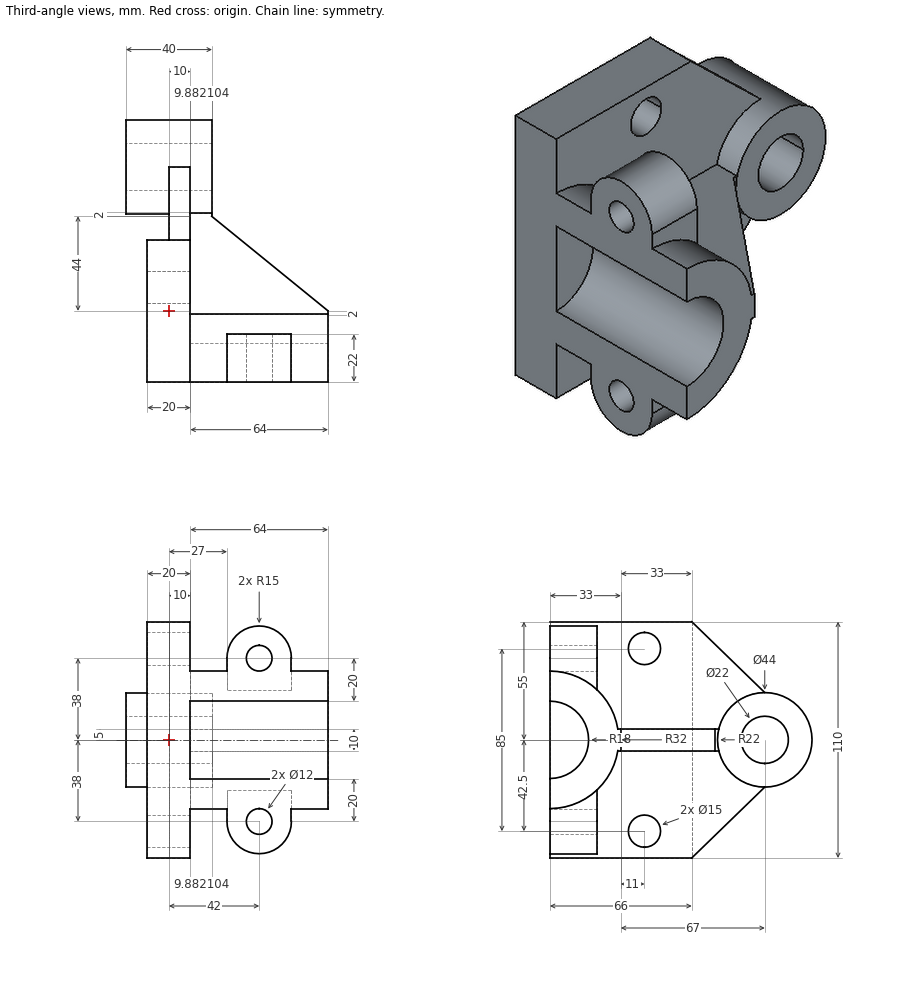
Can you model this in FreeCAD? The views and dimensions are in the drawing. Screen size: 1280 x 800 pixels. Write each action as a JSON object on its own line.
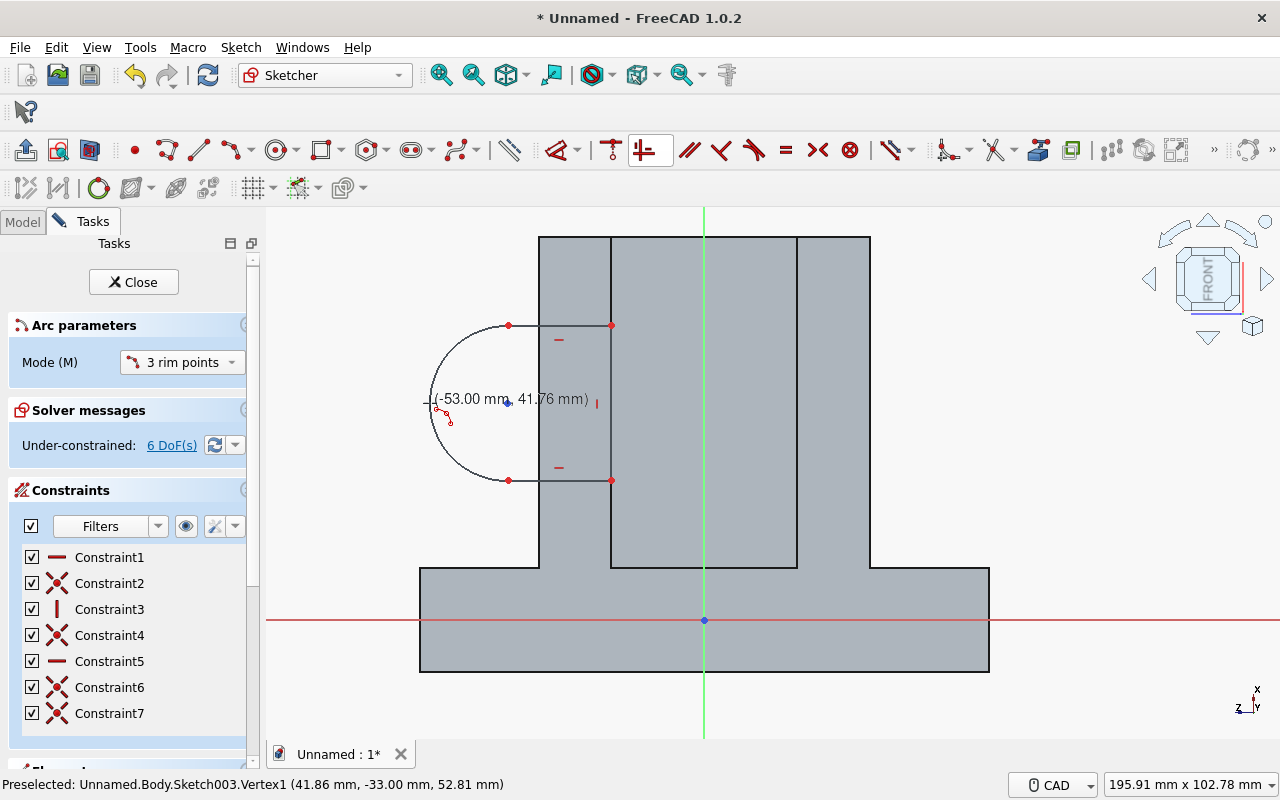
{"action": "left_click", "coordinate": [168, 150]}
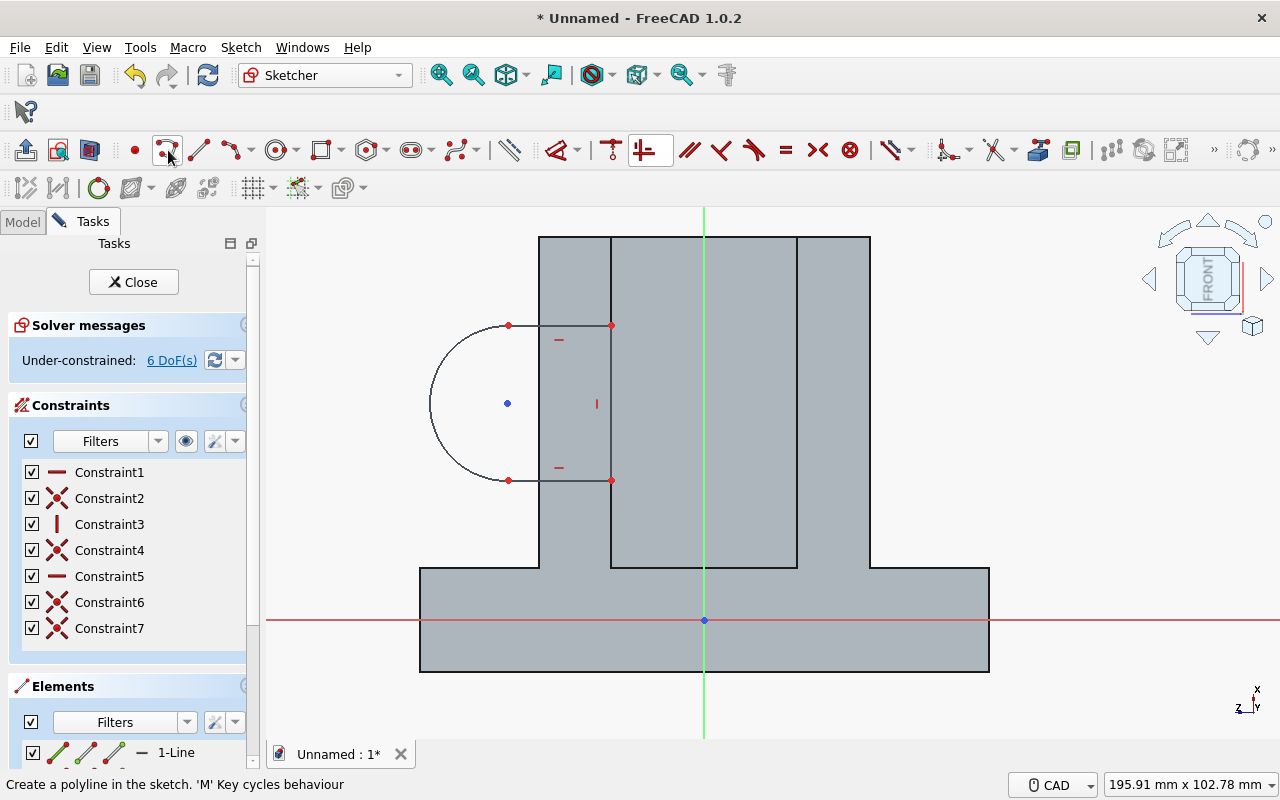
{"action": "left_click", "coordinate": [901, 325]}
{"action": "left_click", "coordinate": [797, 325]}
{"action": "left_click", "coordinate": [797, 480]}
{"action": "left_click", "coordinate": [901, 480]}
{"action": "right_click", "coordinate": [901, 480]}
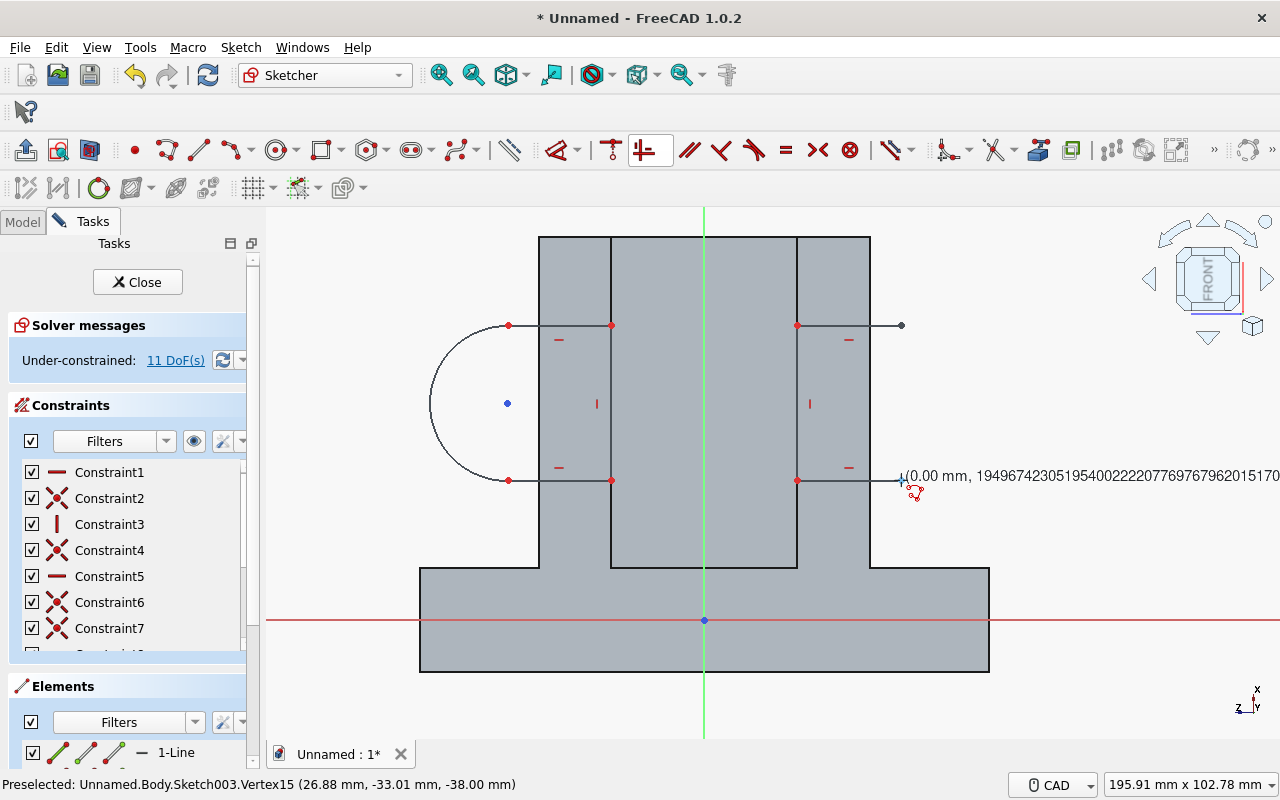
{"action": "left_click", "coordinate": [232, 150]}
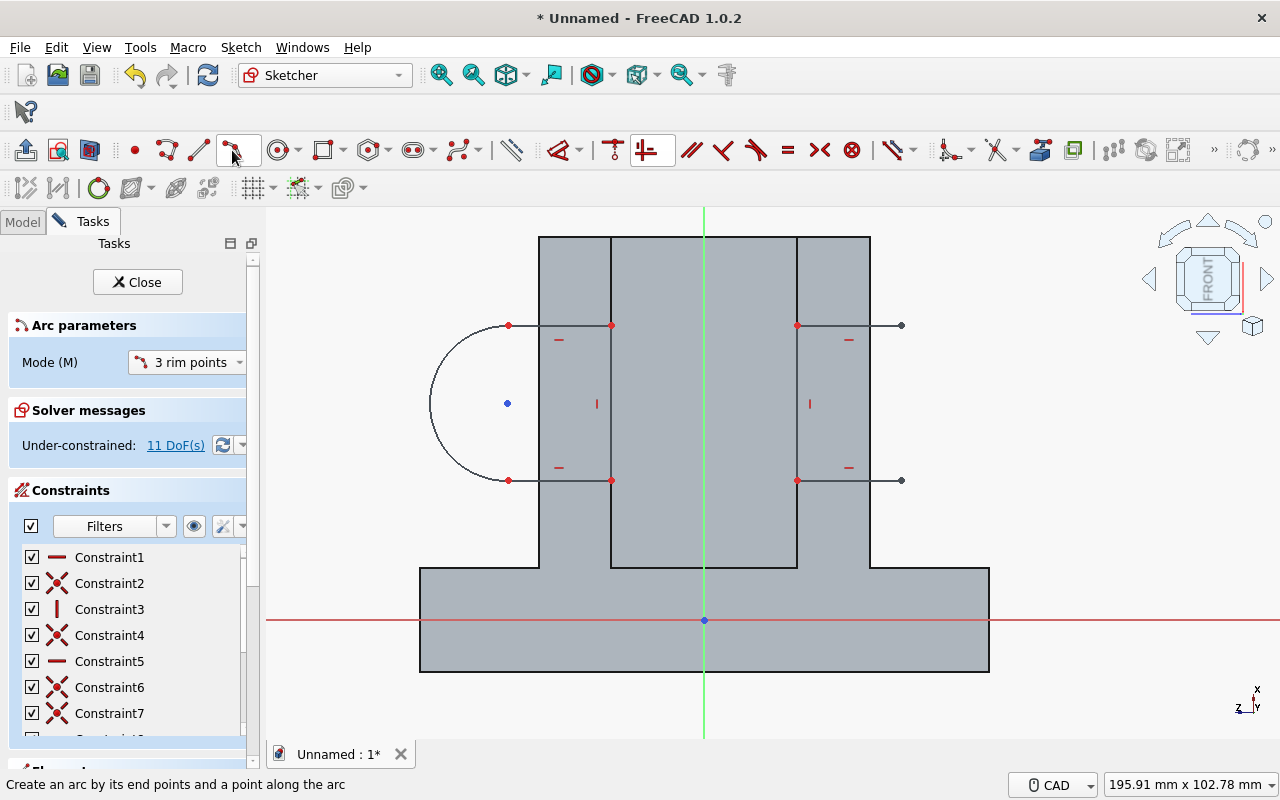
{"action": "left_click", "coordinate": [901, 481]}
{"action": "left_click", "coordinate": [901, 326]}
{"action": "left_click", "coordinate": [979, 403]}
{"action": "key", "text": "Escape"}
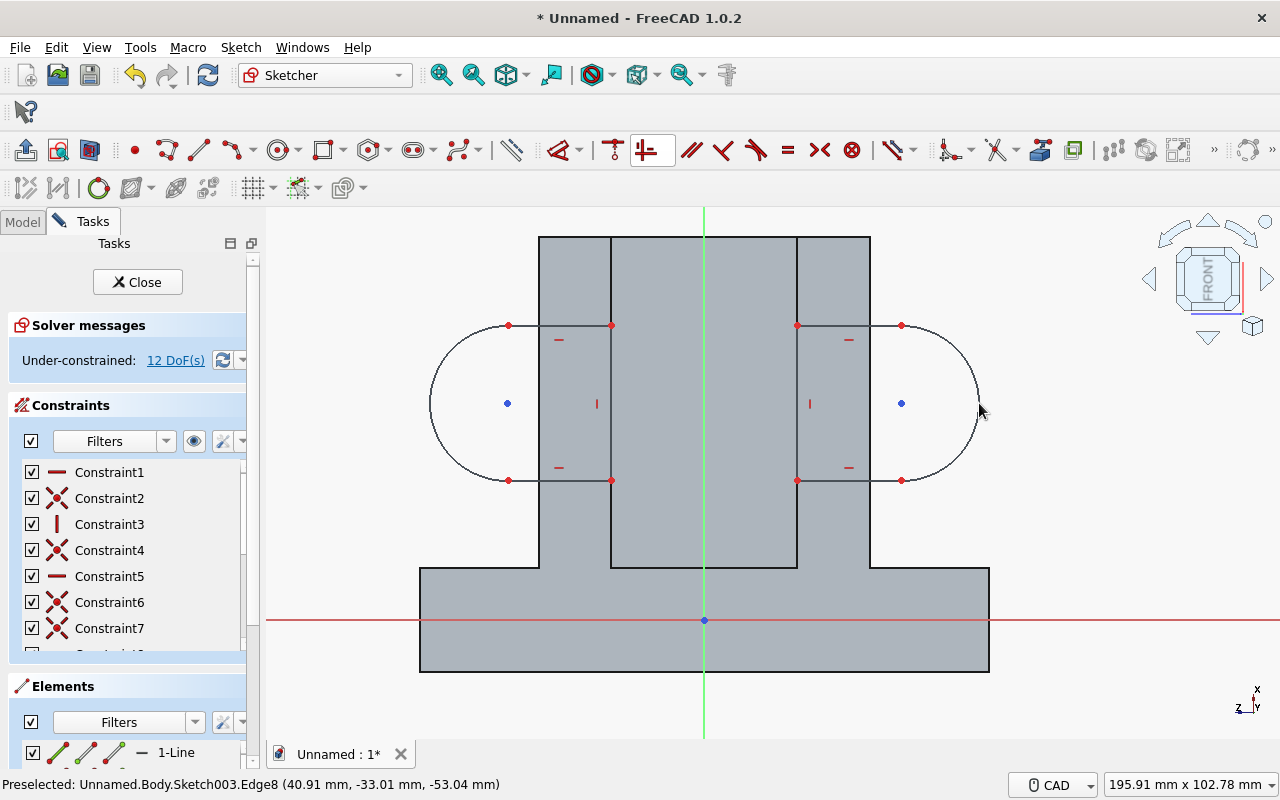
{"action": "left_click", "coordinate": [539, 481]}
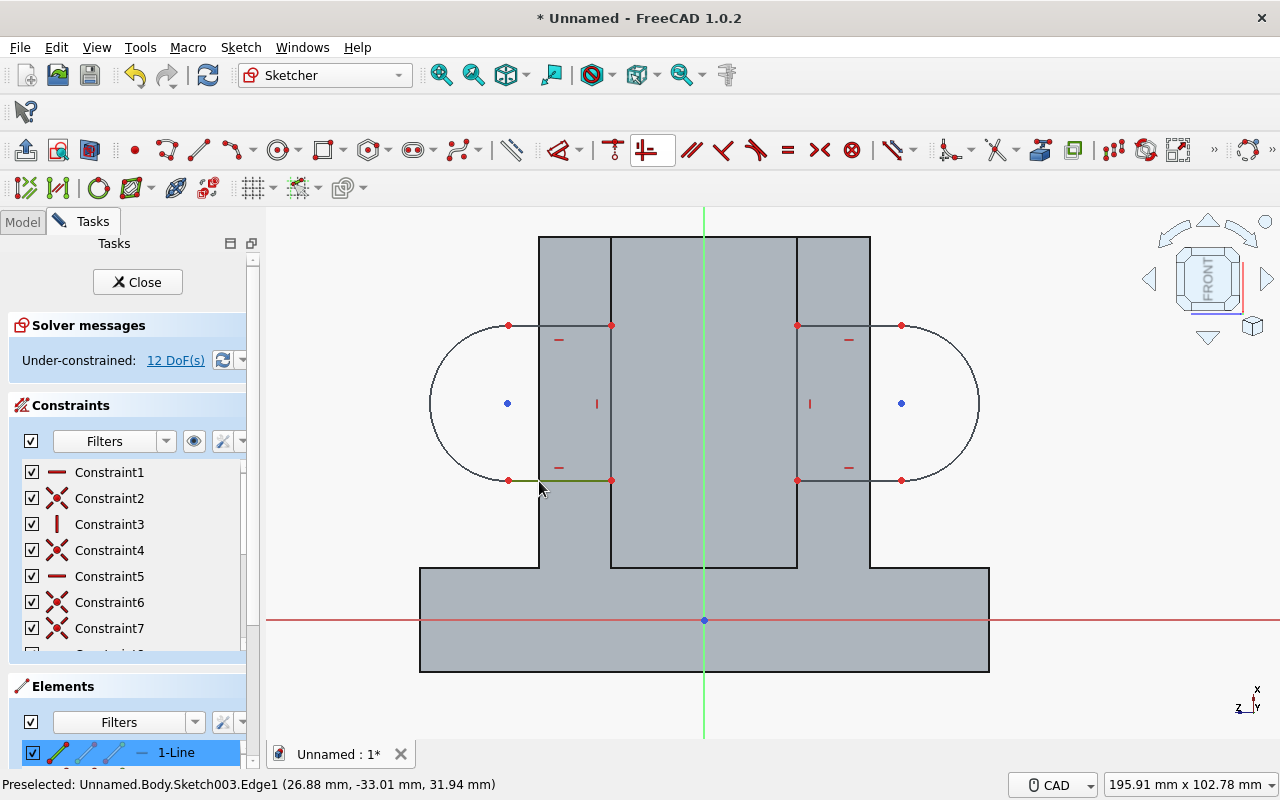
{"action": "left_click", "coordinate": [445, 358]}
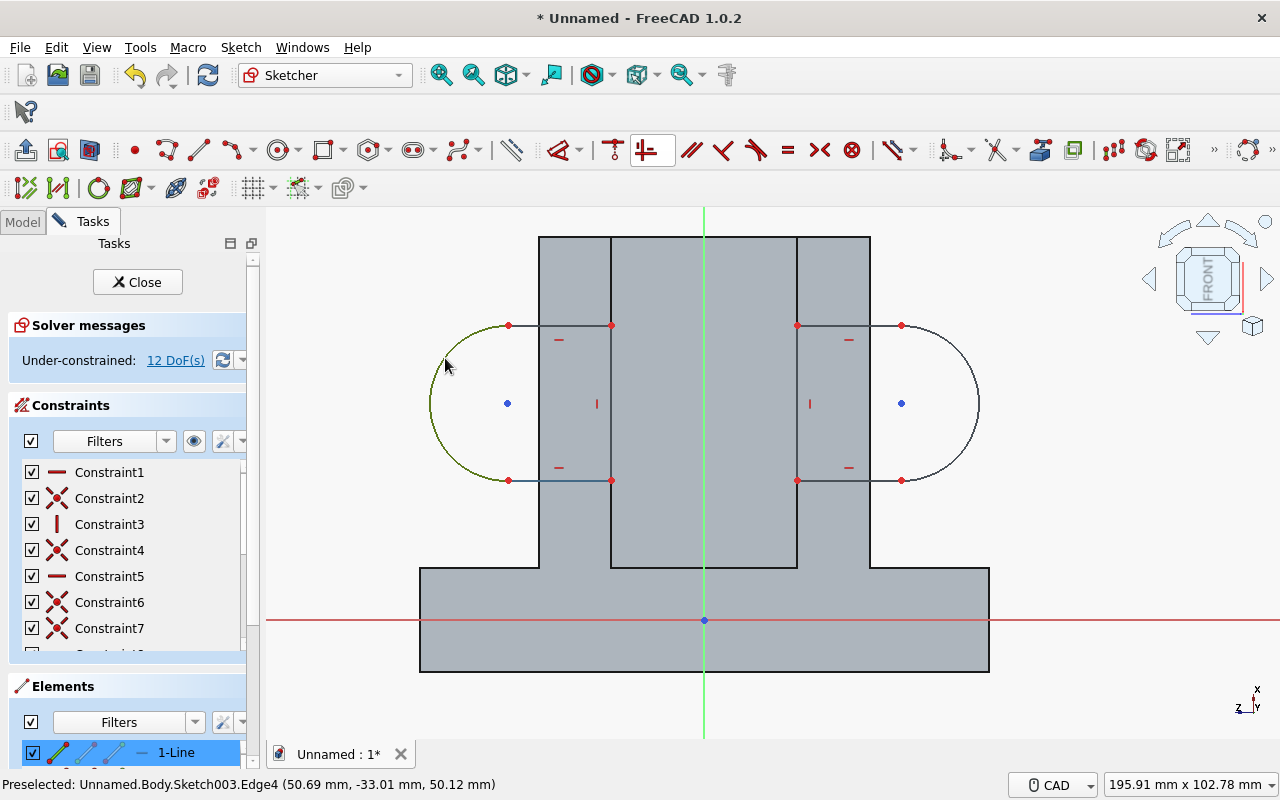
{"action": "left_click", "coordinate": [756, 150]}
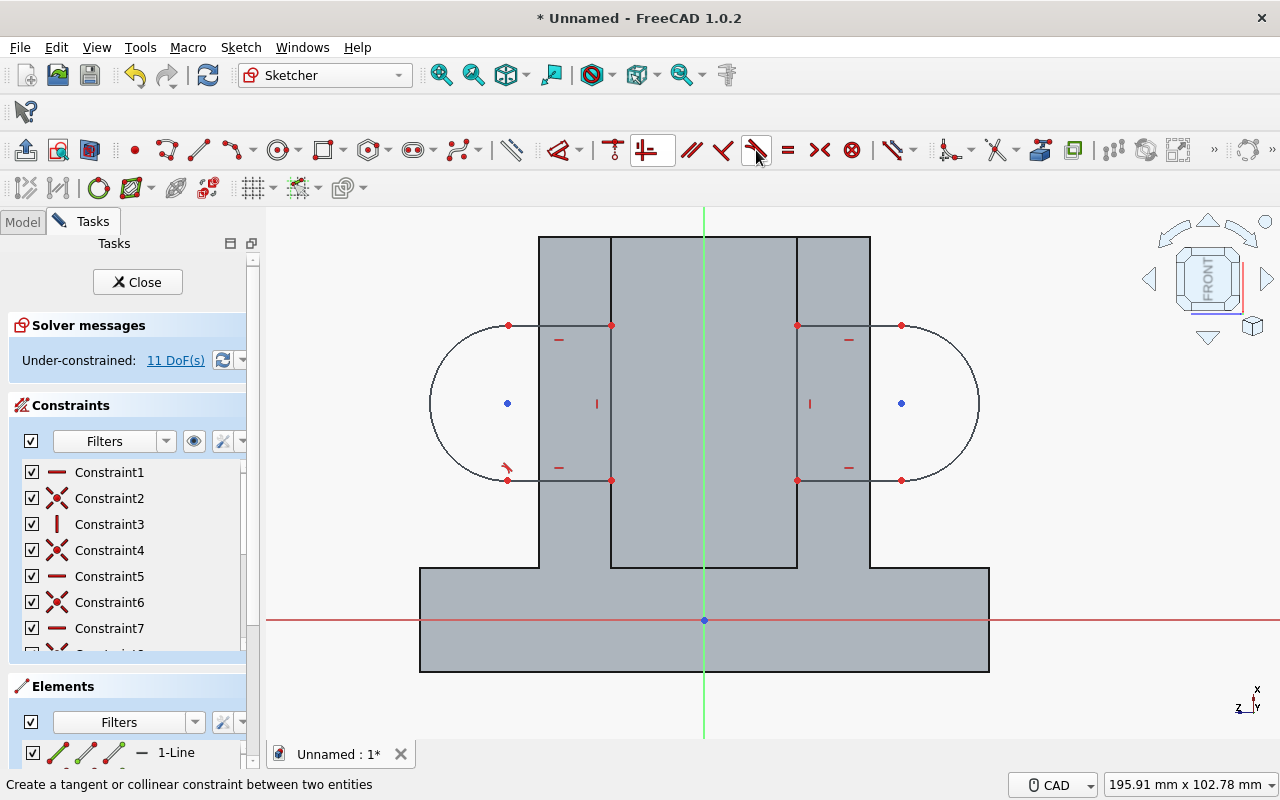
{"action": "left_click", "coordinate": [580, 326]}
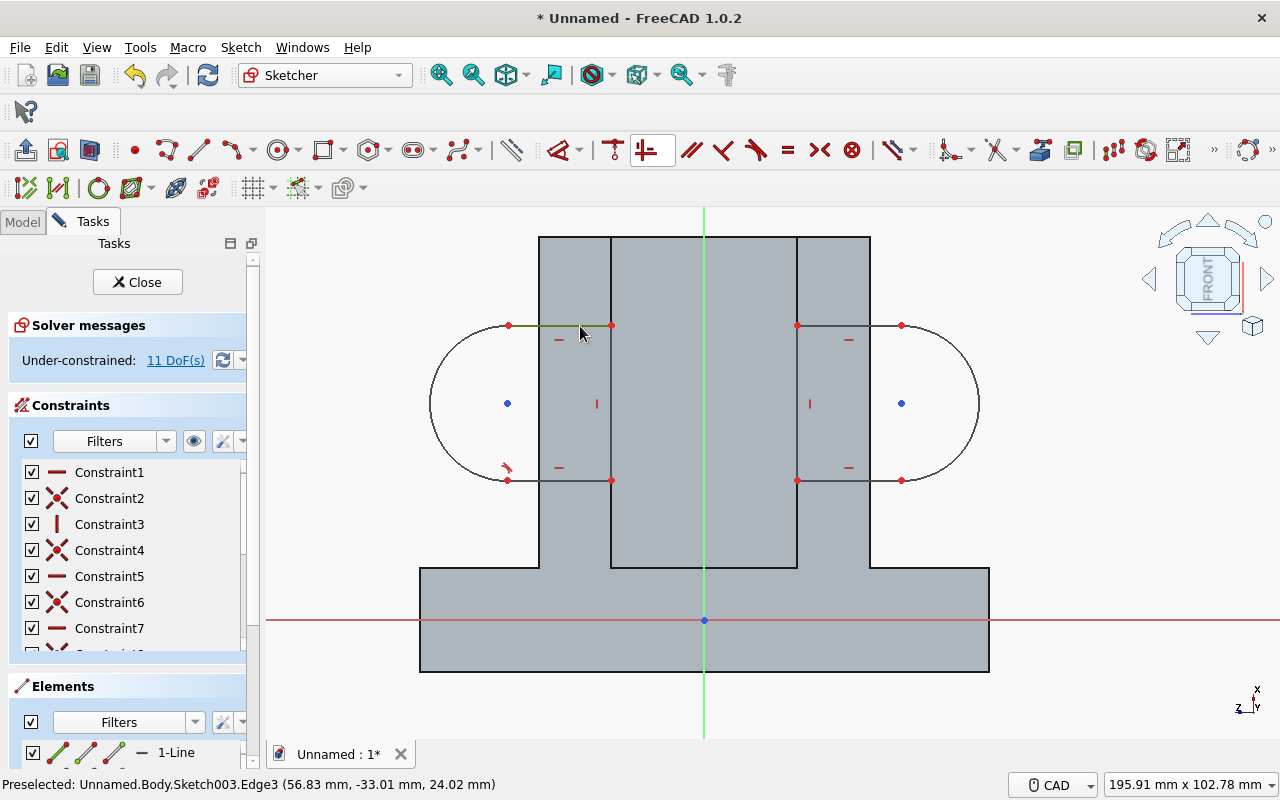
{"action": "left_click", "coordinate": [445, 358]}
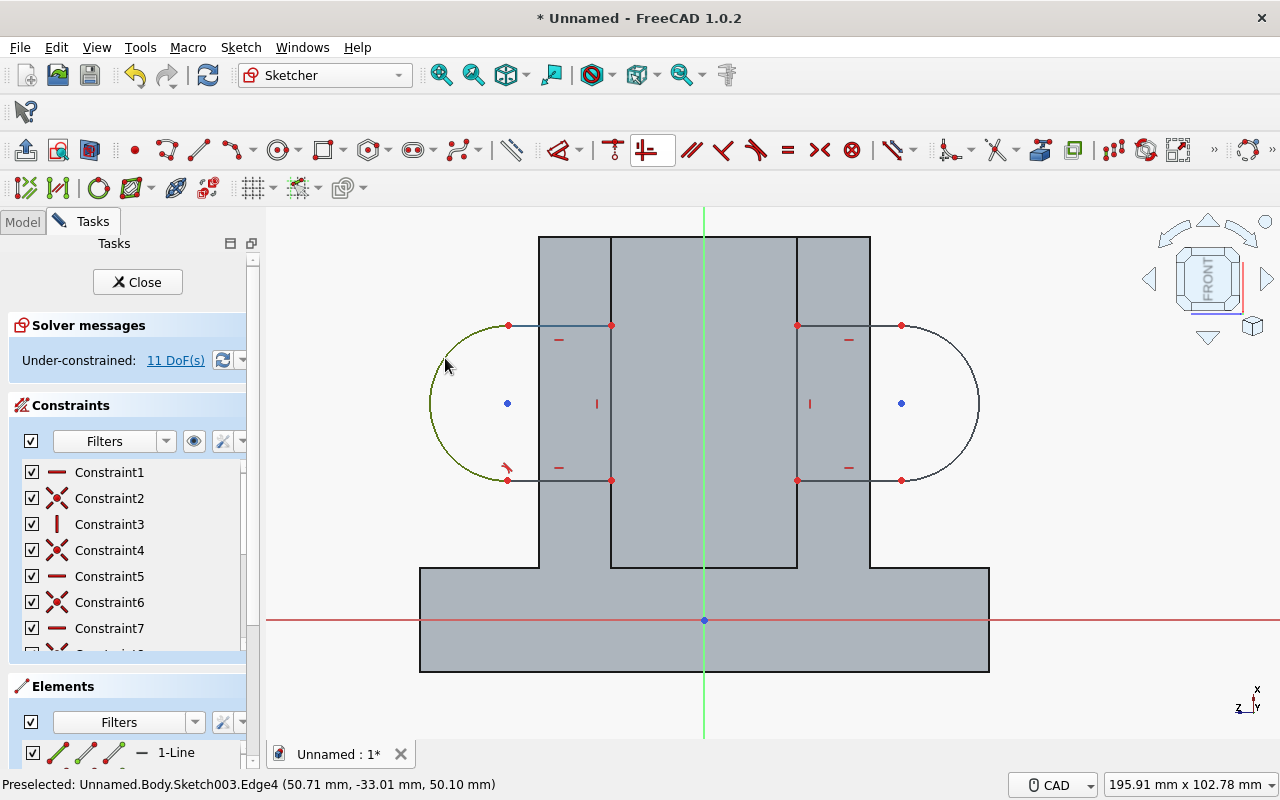
{"action": "left_click", "coordinate": [756, 150]}